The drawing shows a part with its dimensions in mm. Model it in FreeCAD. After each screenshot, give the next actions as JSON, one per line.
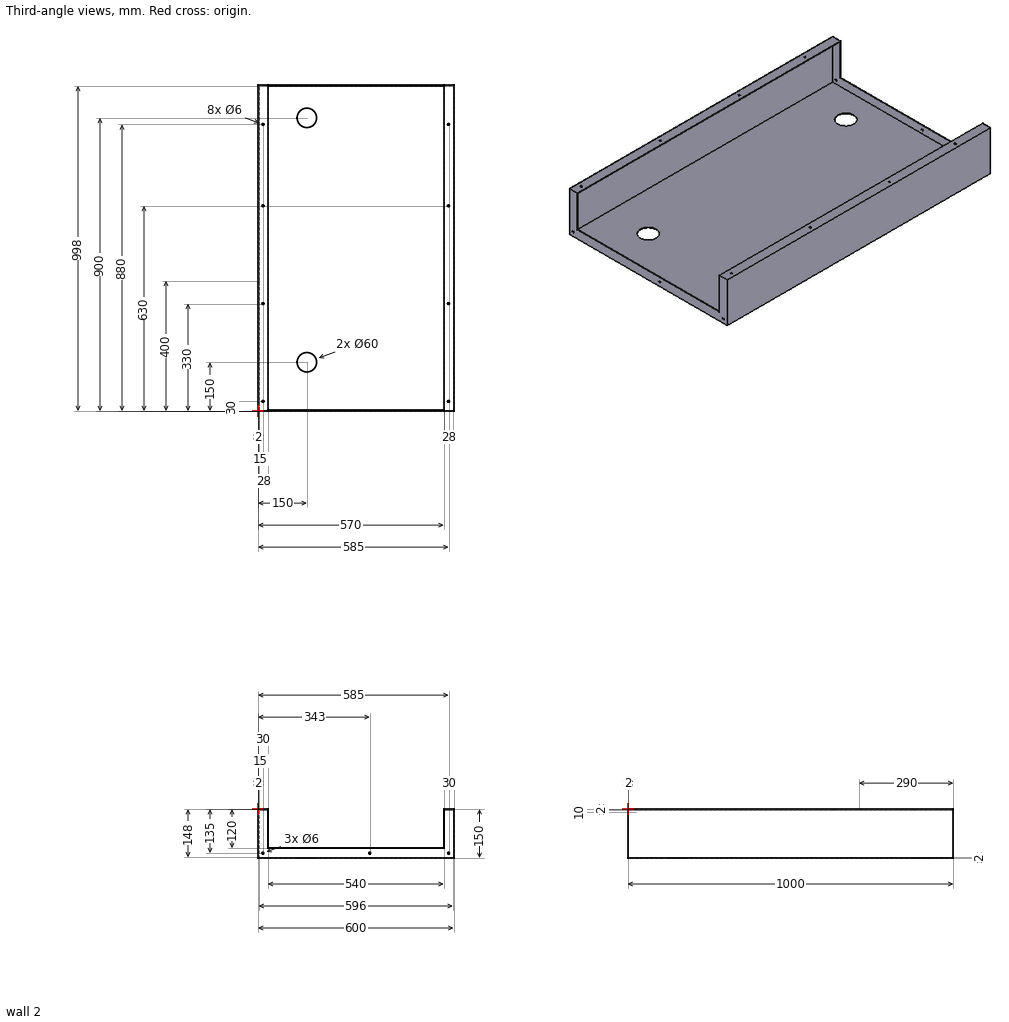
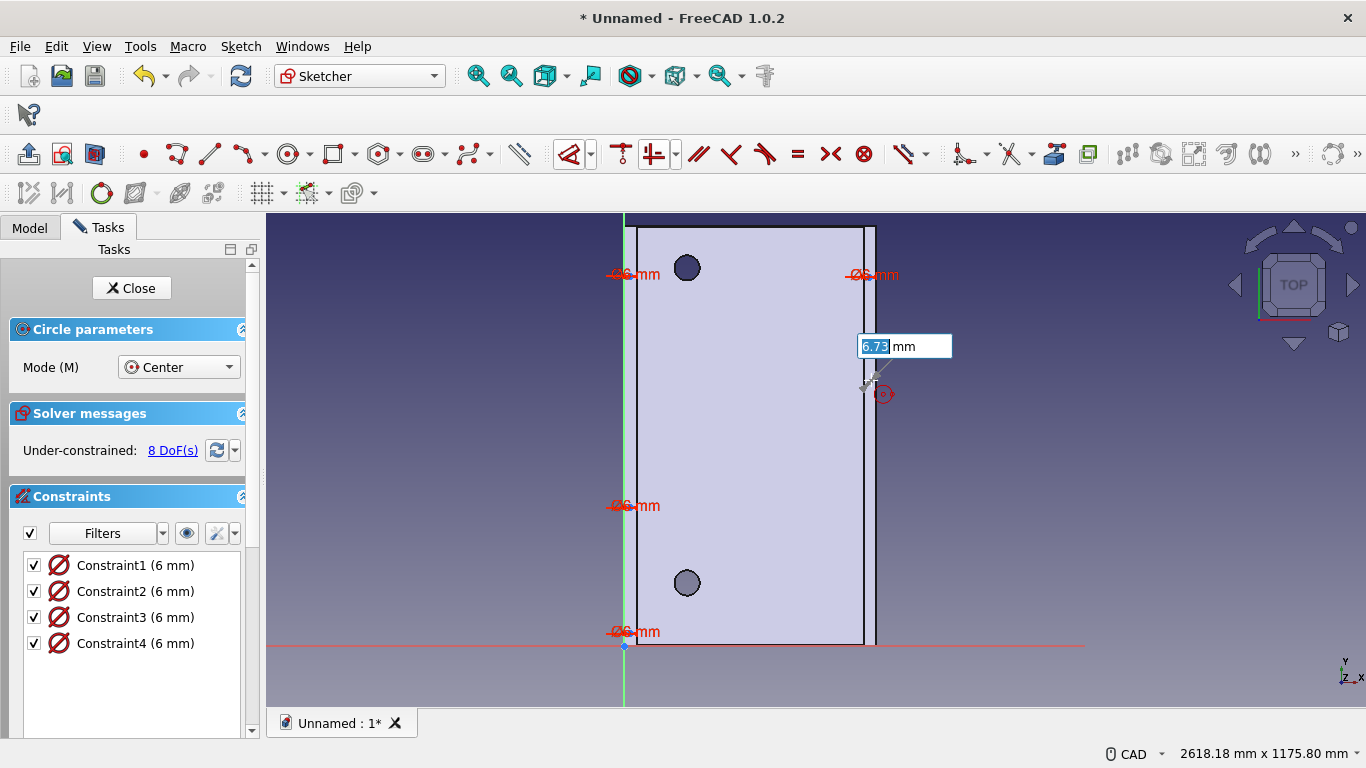
{"action": "type", "text": "6"}
{"action": "key", "text": "Return"}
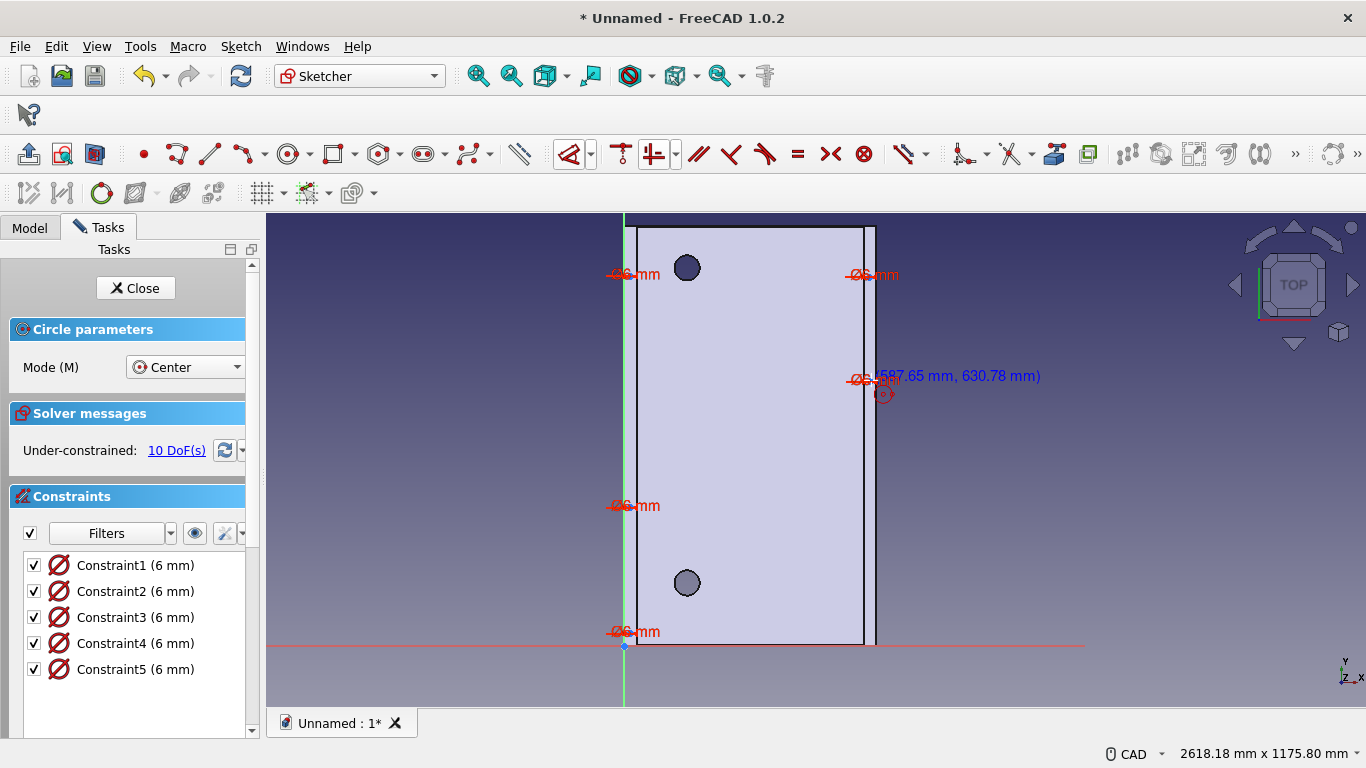
{"action": "scroll", "coordinate": [630, 381], "scroll_direction": "up", "scroll_amount": 15}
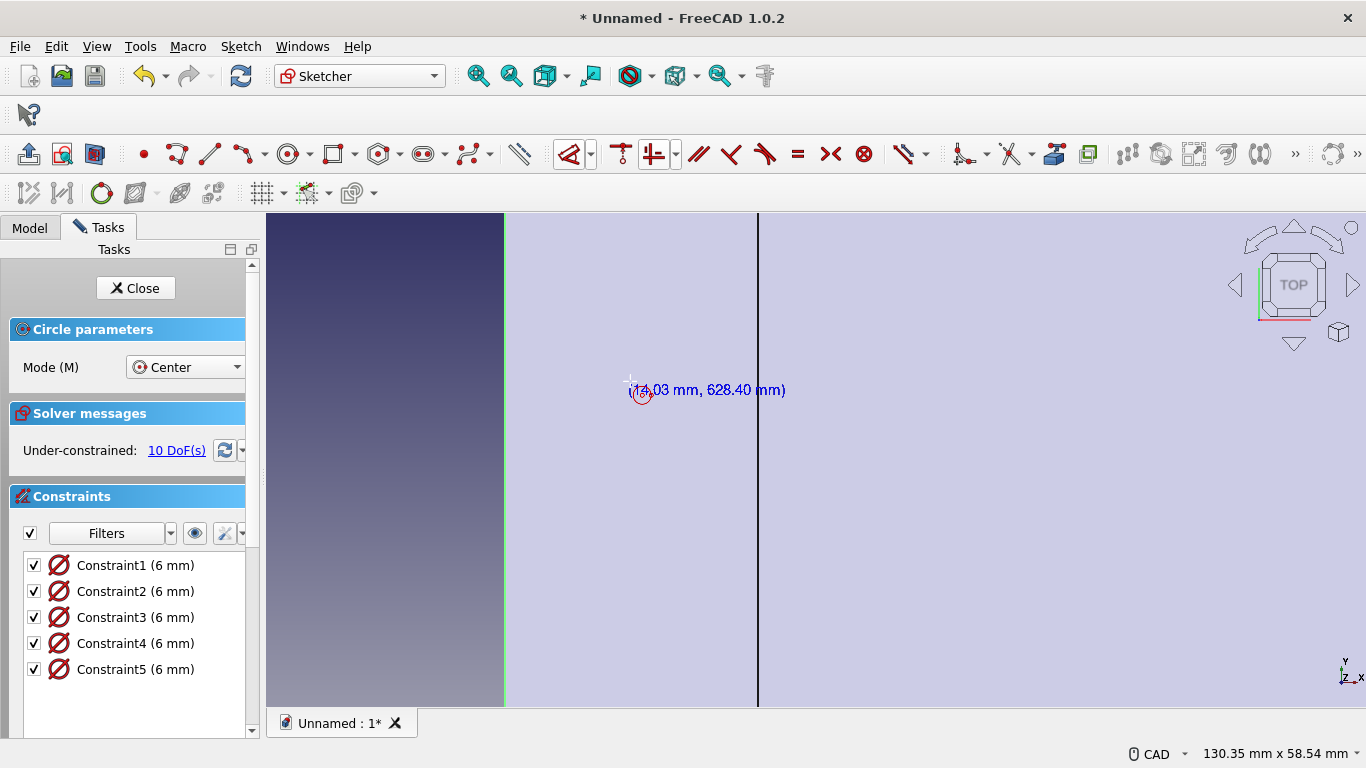
{"action": "scroll", "coordinate": [630, 381], "scroll_direction": "down", "scroll_amount": 15}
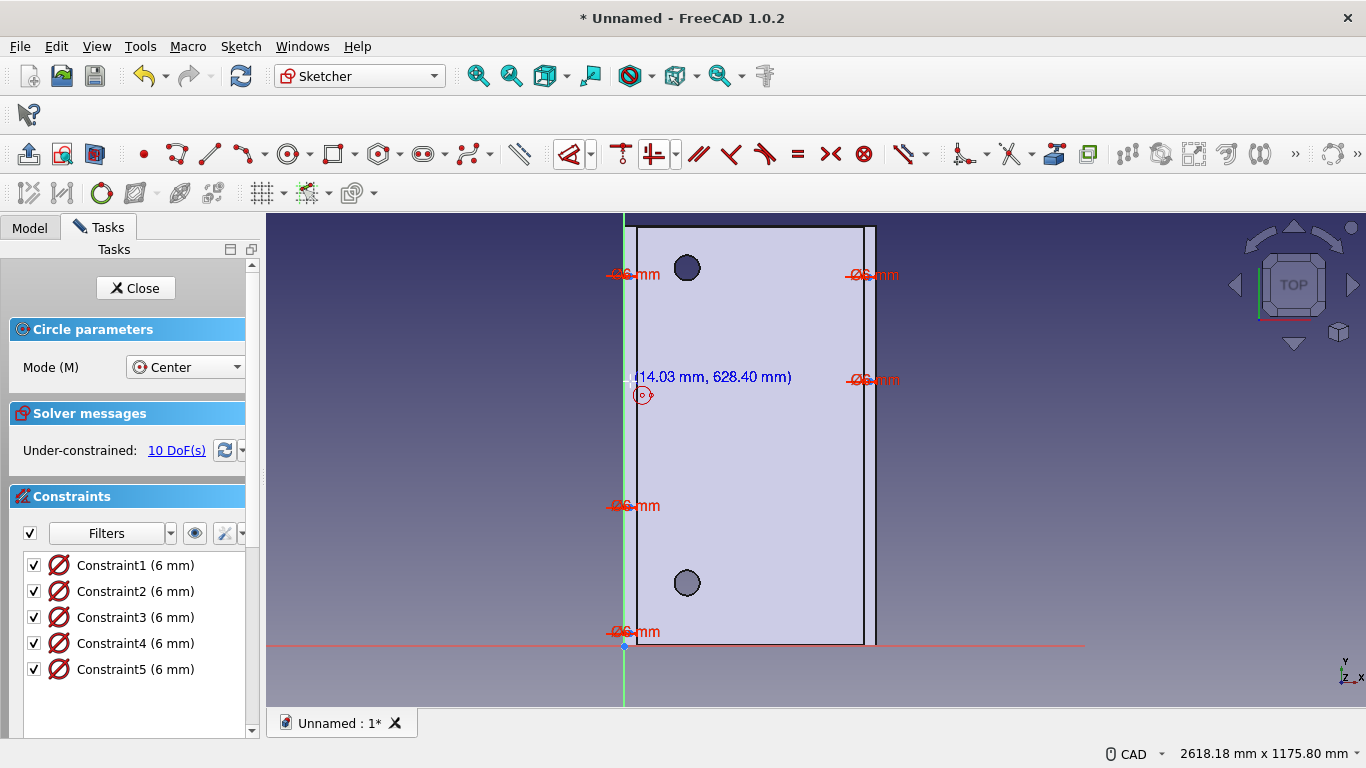
{"action": "scroll", "coordinate": [630, 381], "scroll_direction": "up", "scroll_amount": 5}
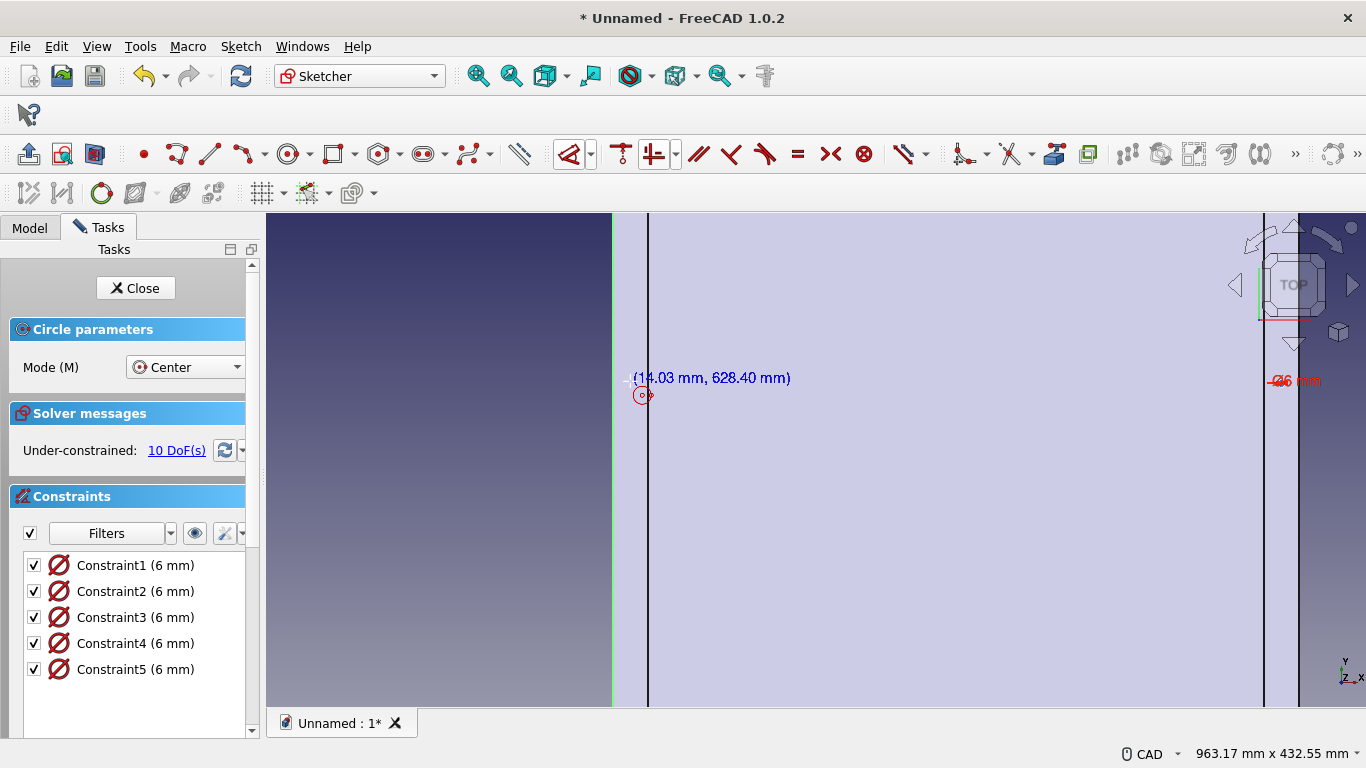
{"action": "left_click", "coordinate": [631, 381]}
{"action": "mouse_move", "coordinate": [633, 379]}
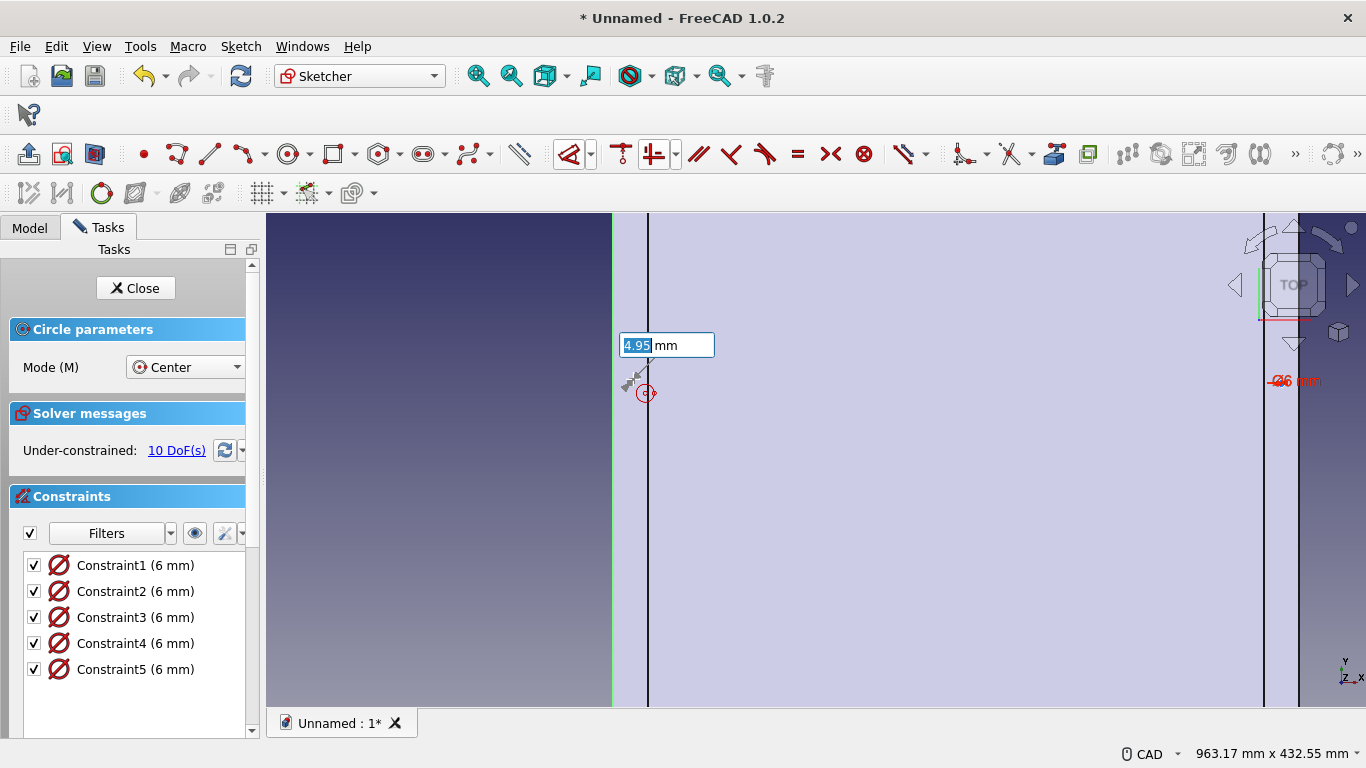
{"action": "type", "text": "6"}
{"action": "key", "text": "Return"}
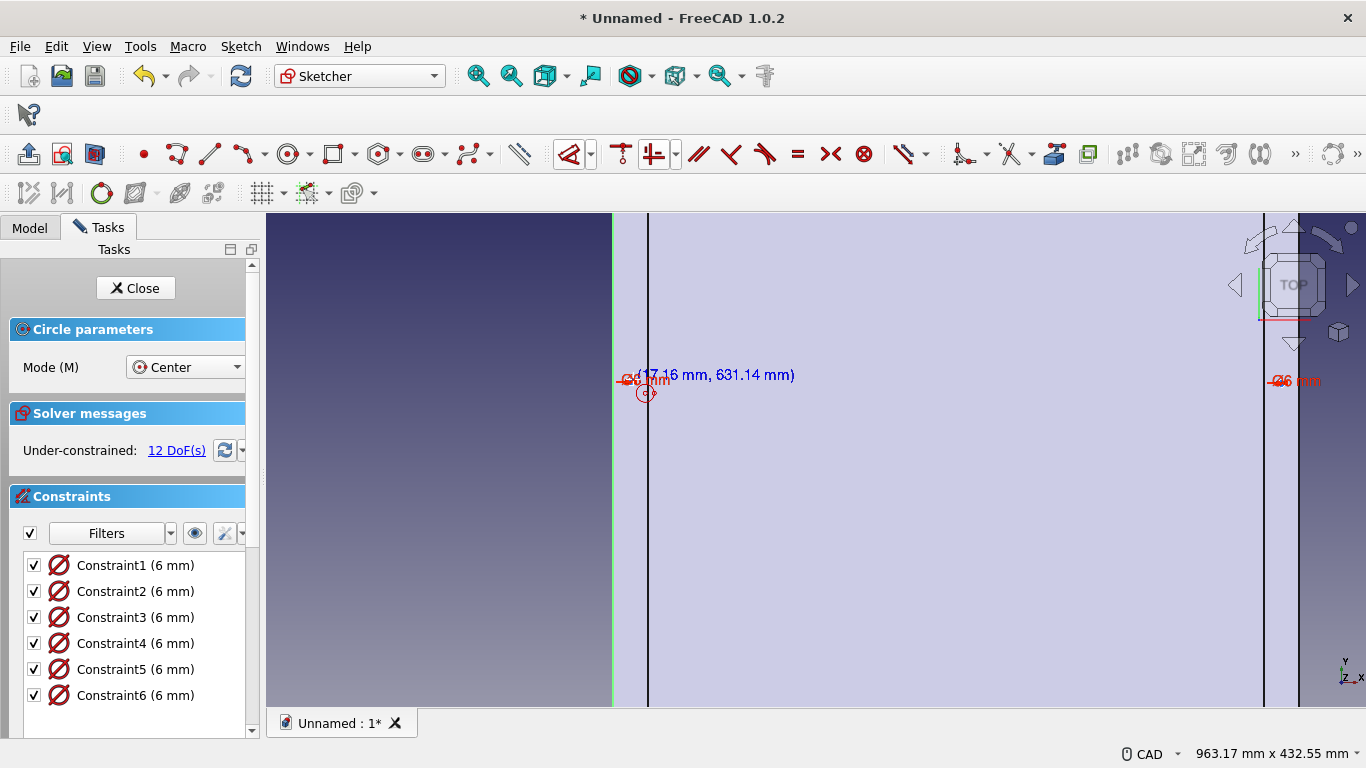
{"action": "scroll", "coordinate": [661, 401], "scroll_direction": "down", "scroll_amount": 6}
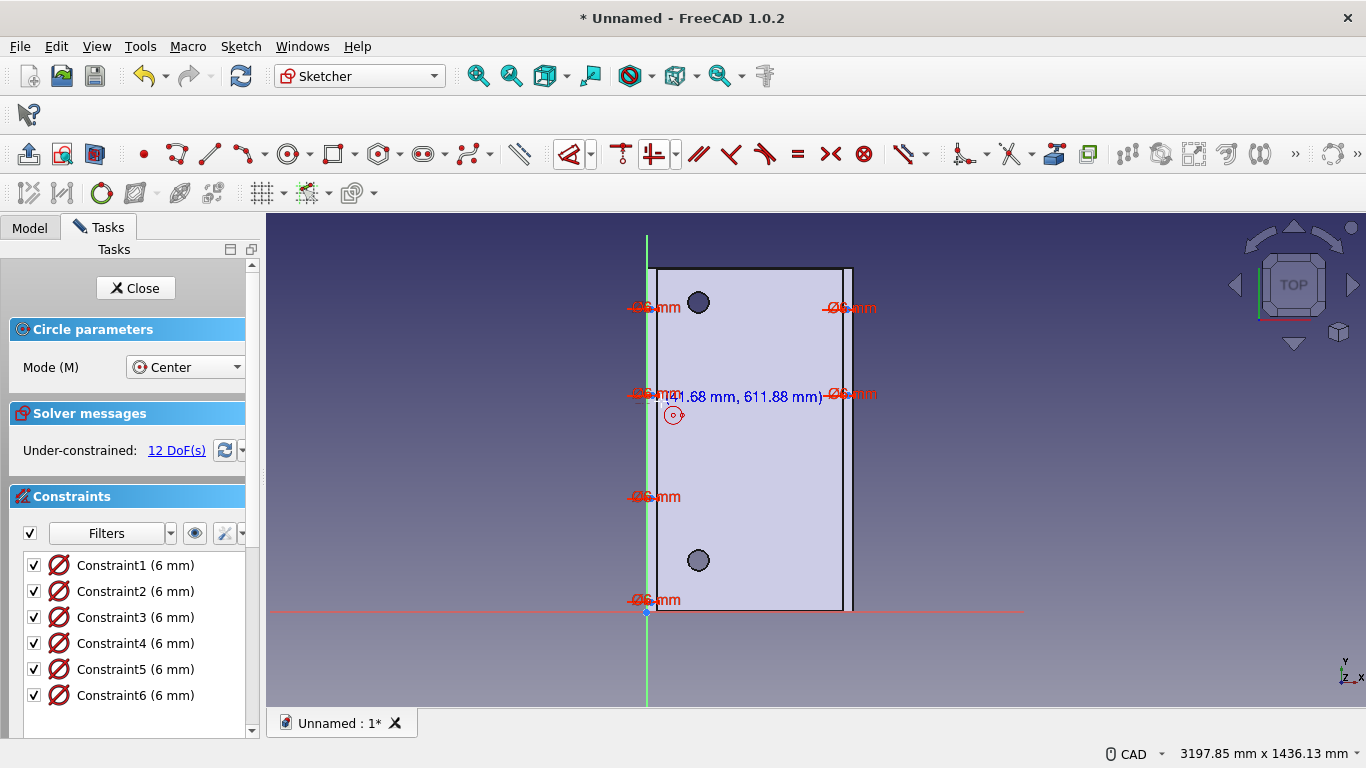
{"action": "scroll", "coordinate": [848, 499], "scroll_direction": "up", "scroll_amount": 16}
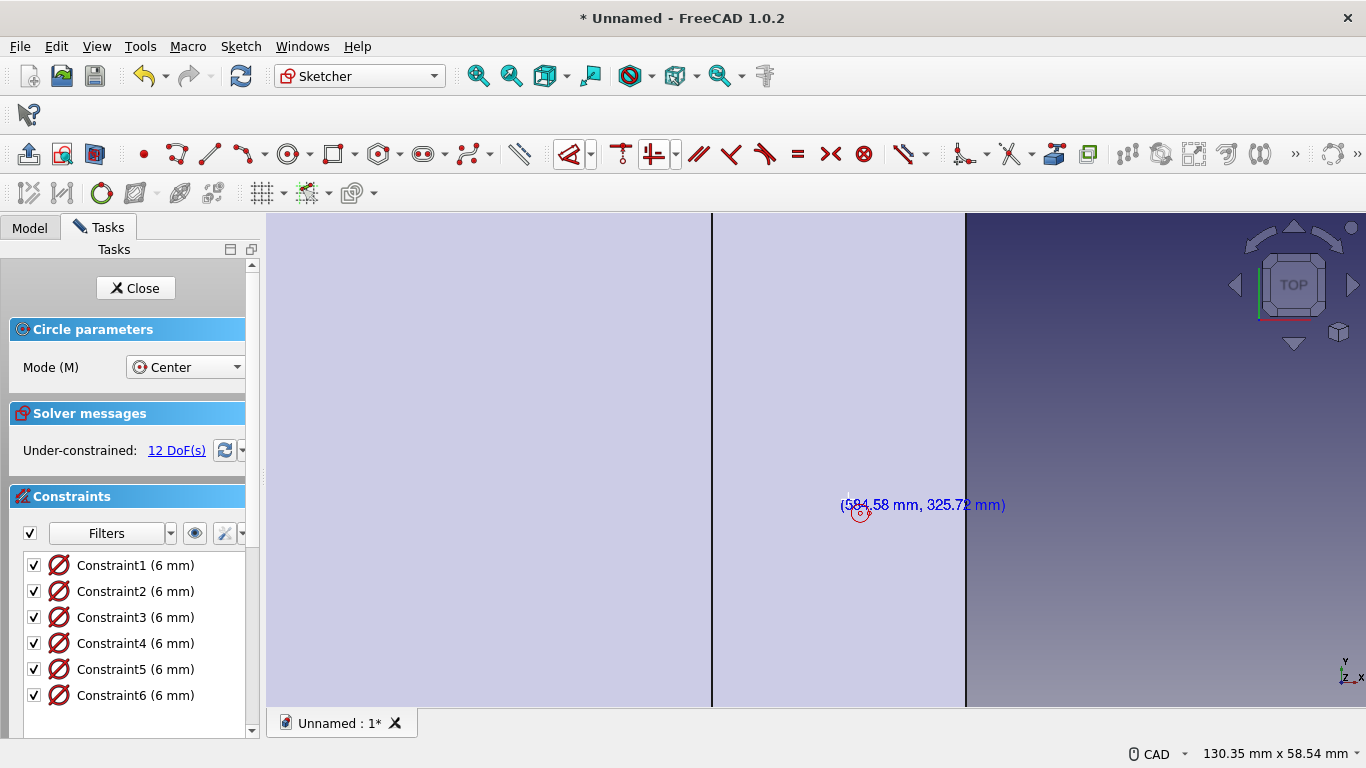
{"action": "scroll", "coordinate": [871, 509], "scroll_direction": "down", "scroll_amount": 15}